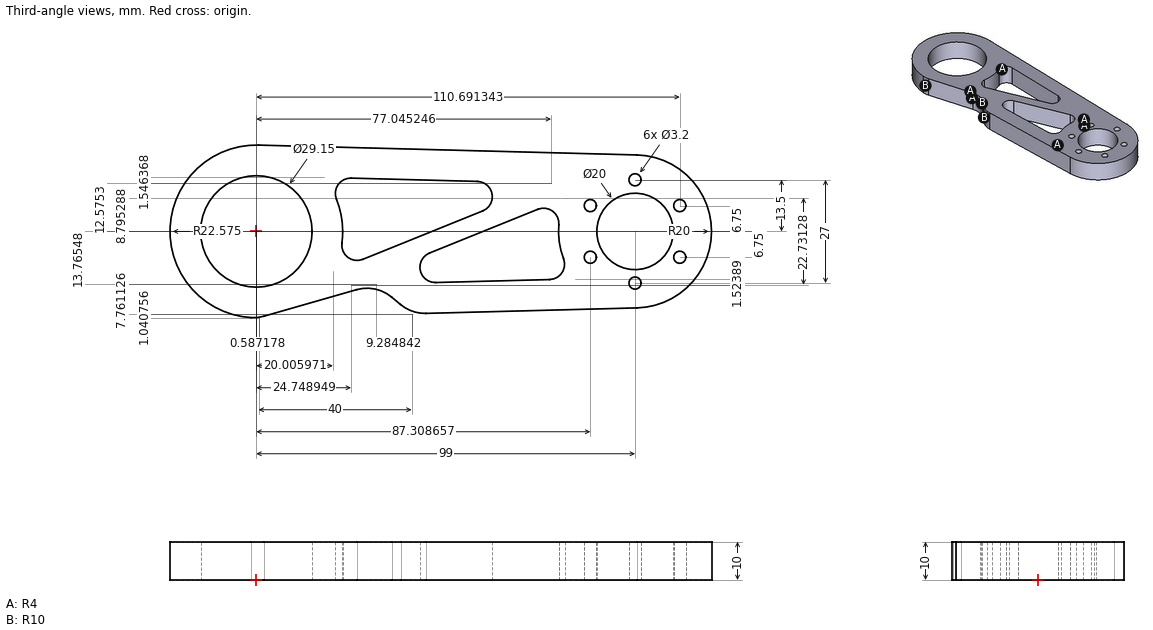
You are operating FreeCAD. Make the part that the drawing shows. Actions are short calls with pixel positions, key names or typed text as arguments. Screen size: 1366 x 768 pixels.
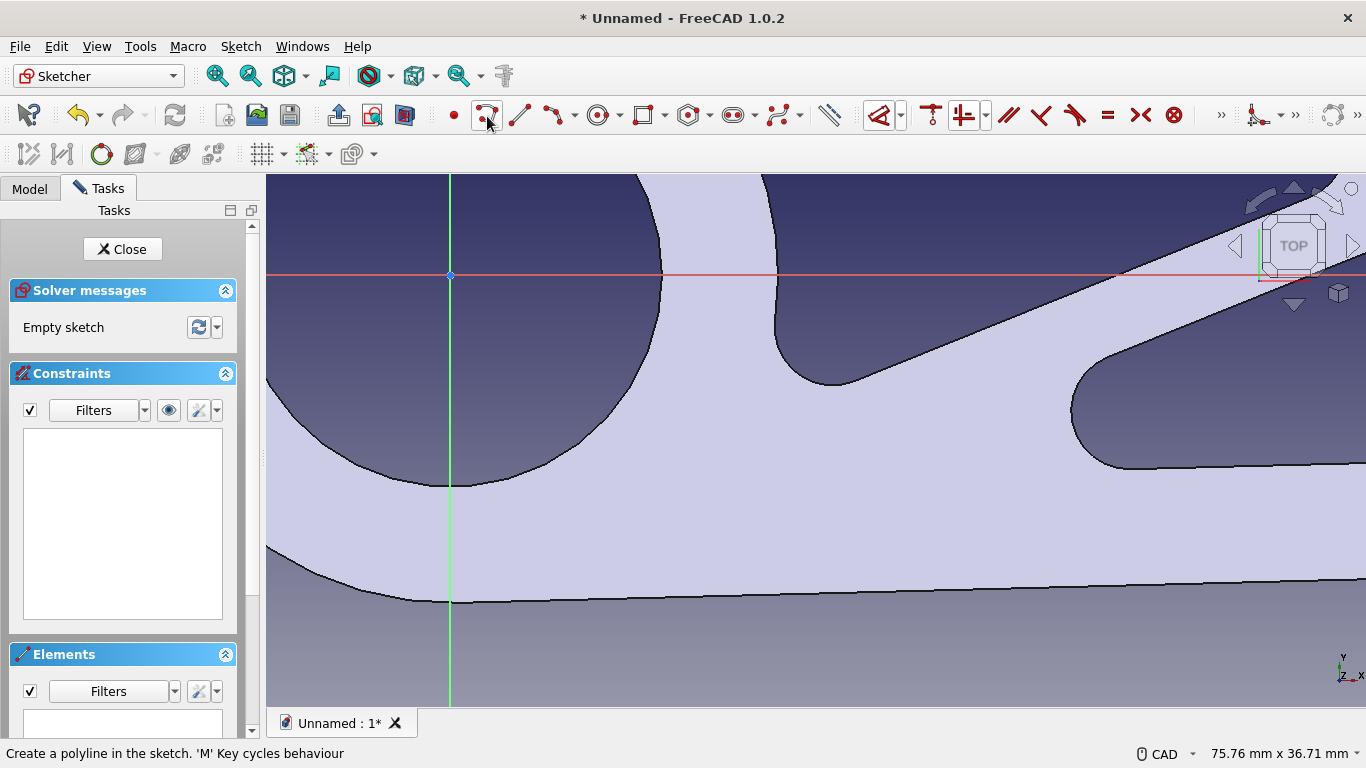
scroll(459, 603, up, 4)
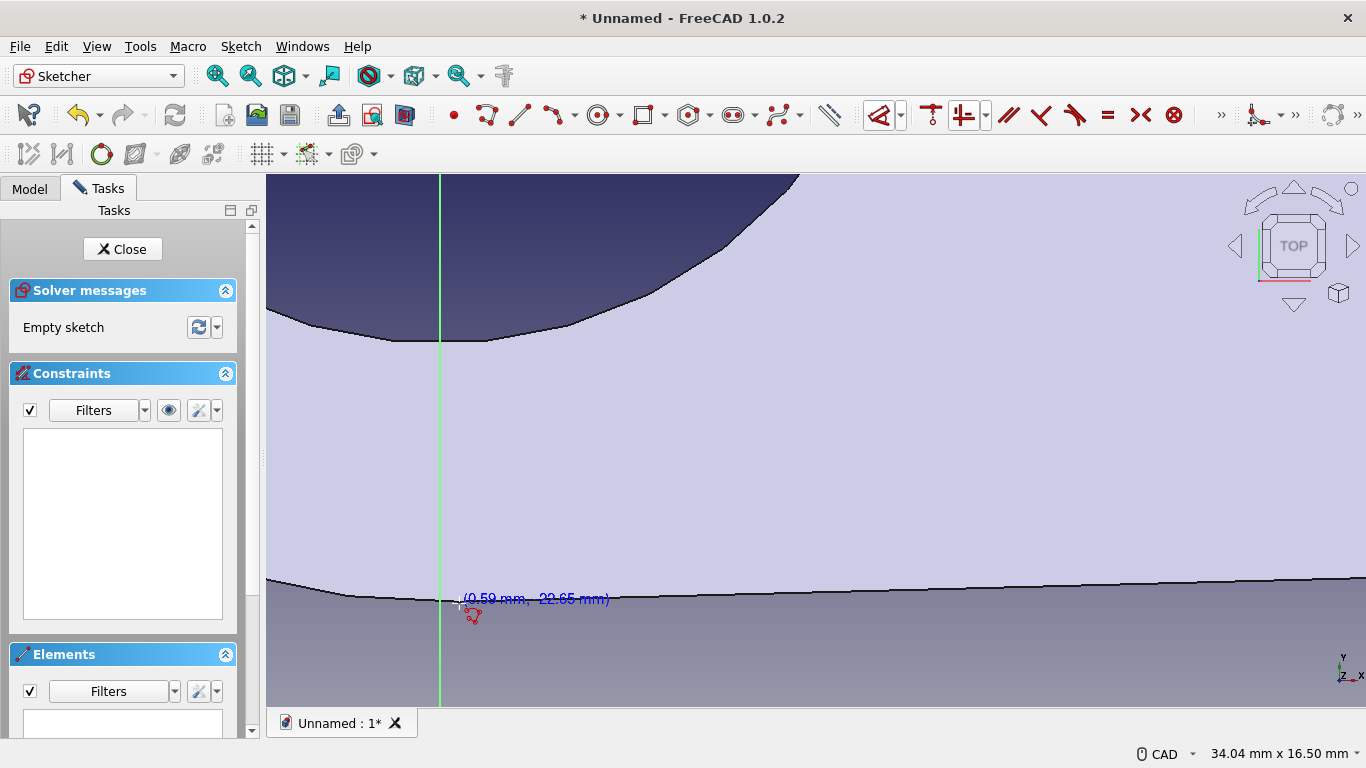
click(459, 602)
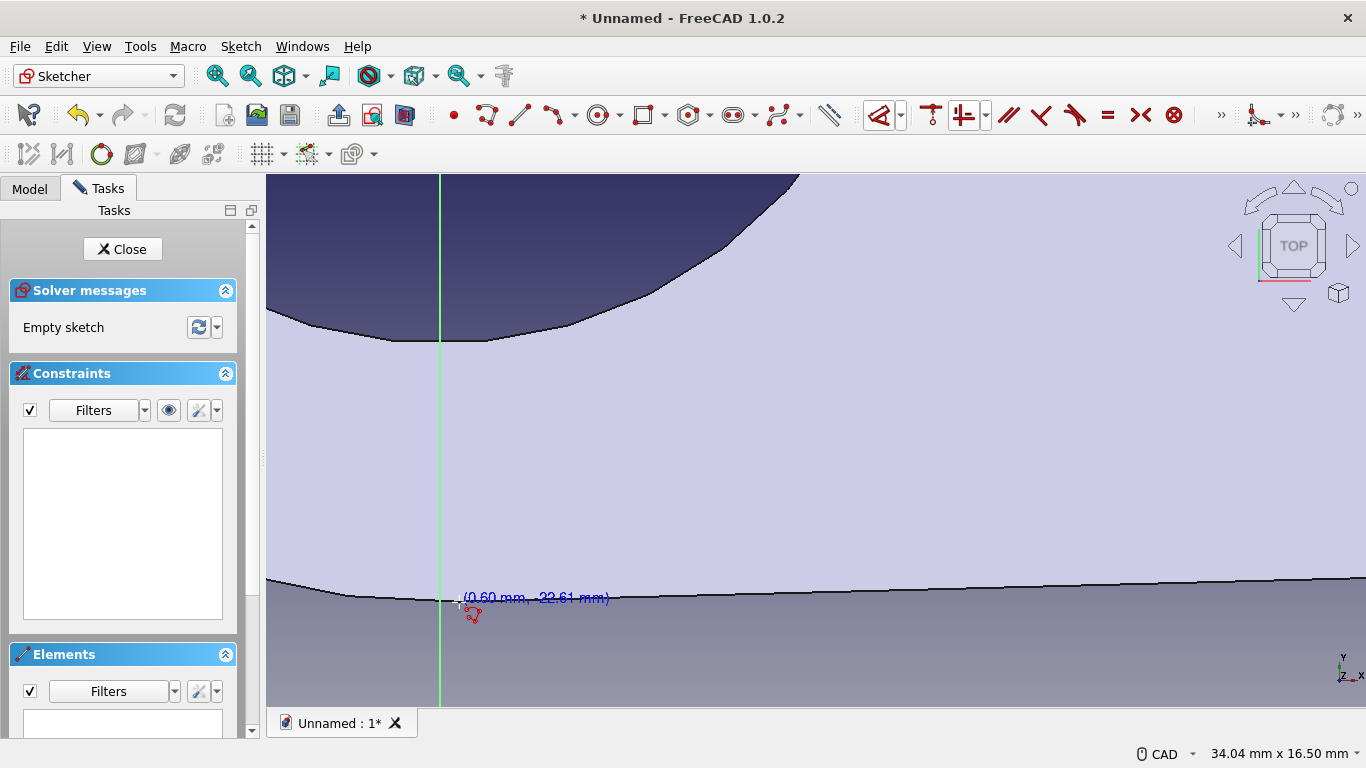
scroll(464, 606, down, 4)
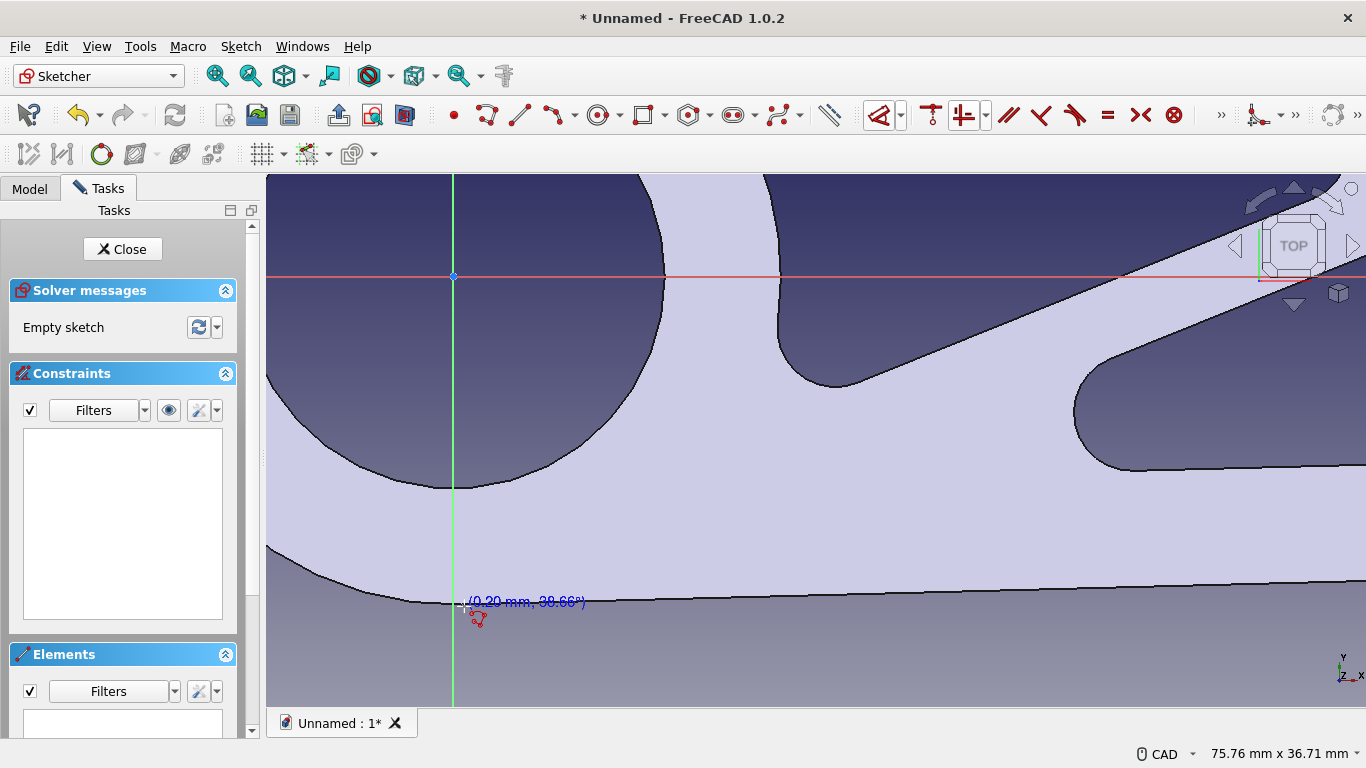
click(1042, 577)
click(908, 477)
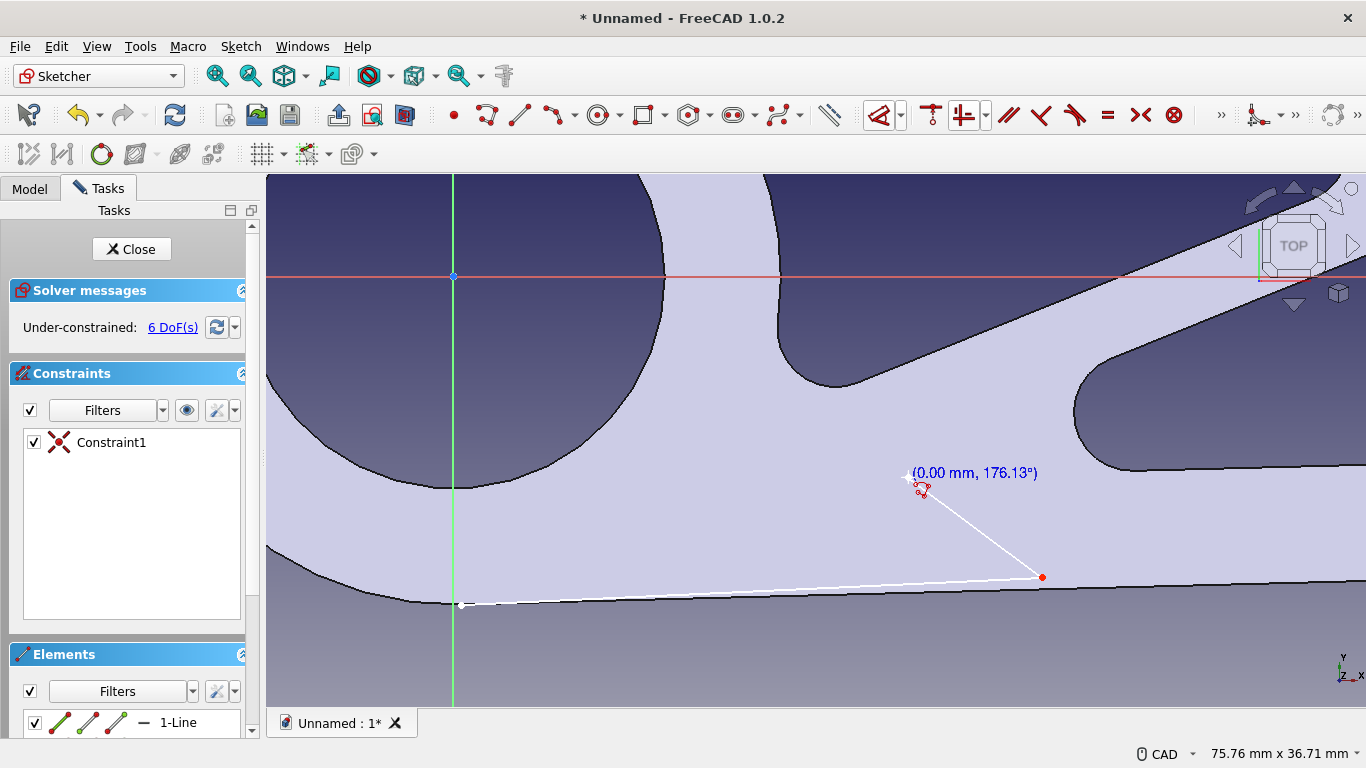
scroll(462, 605, up, 4)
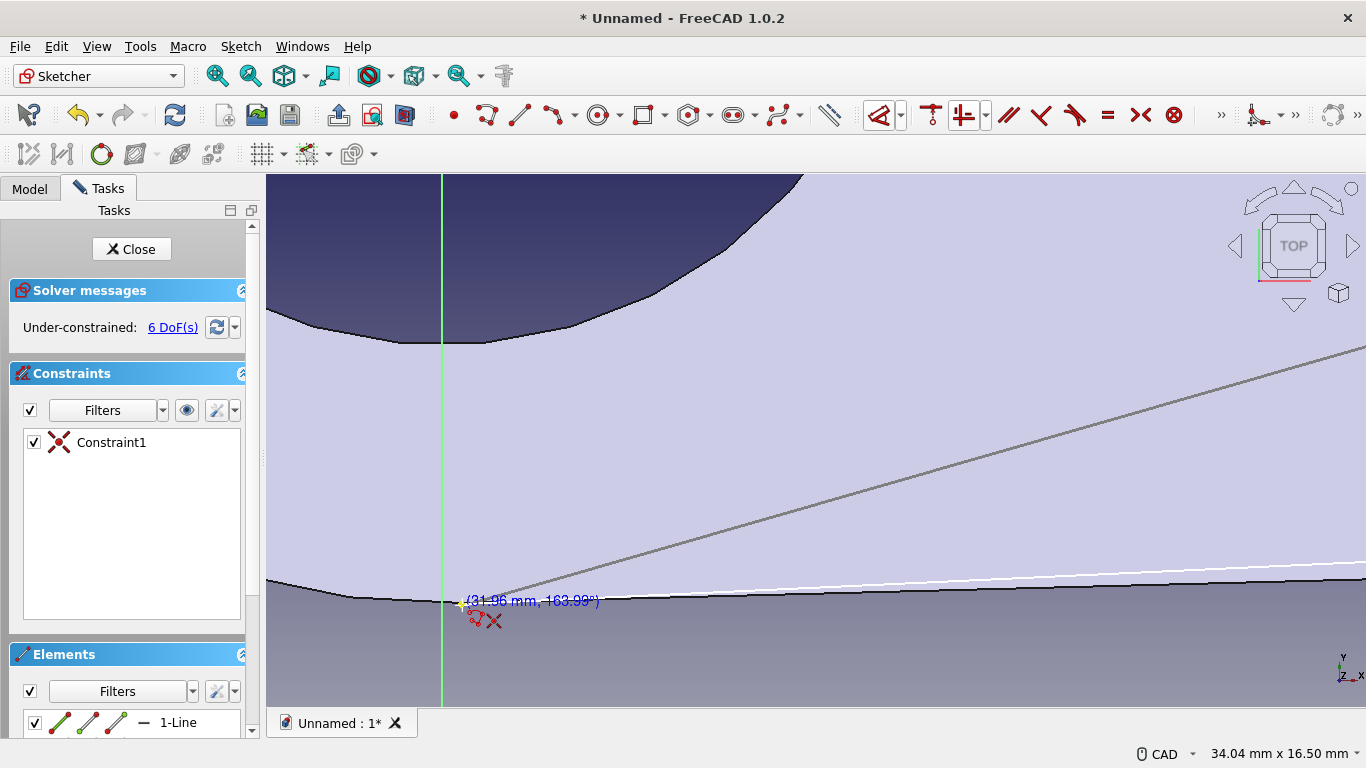
click(461, 604)
key(Escape)
key(Escape)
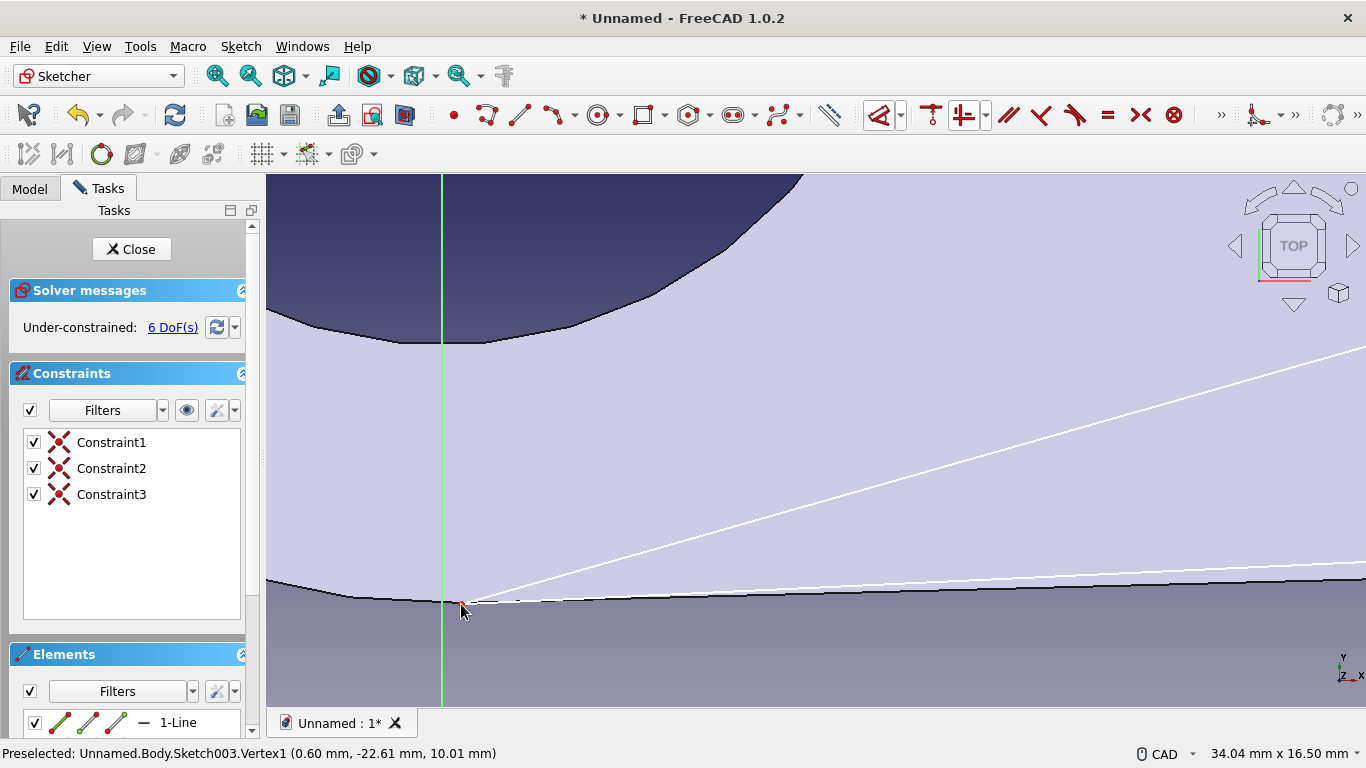
click(849, 586)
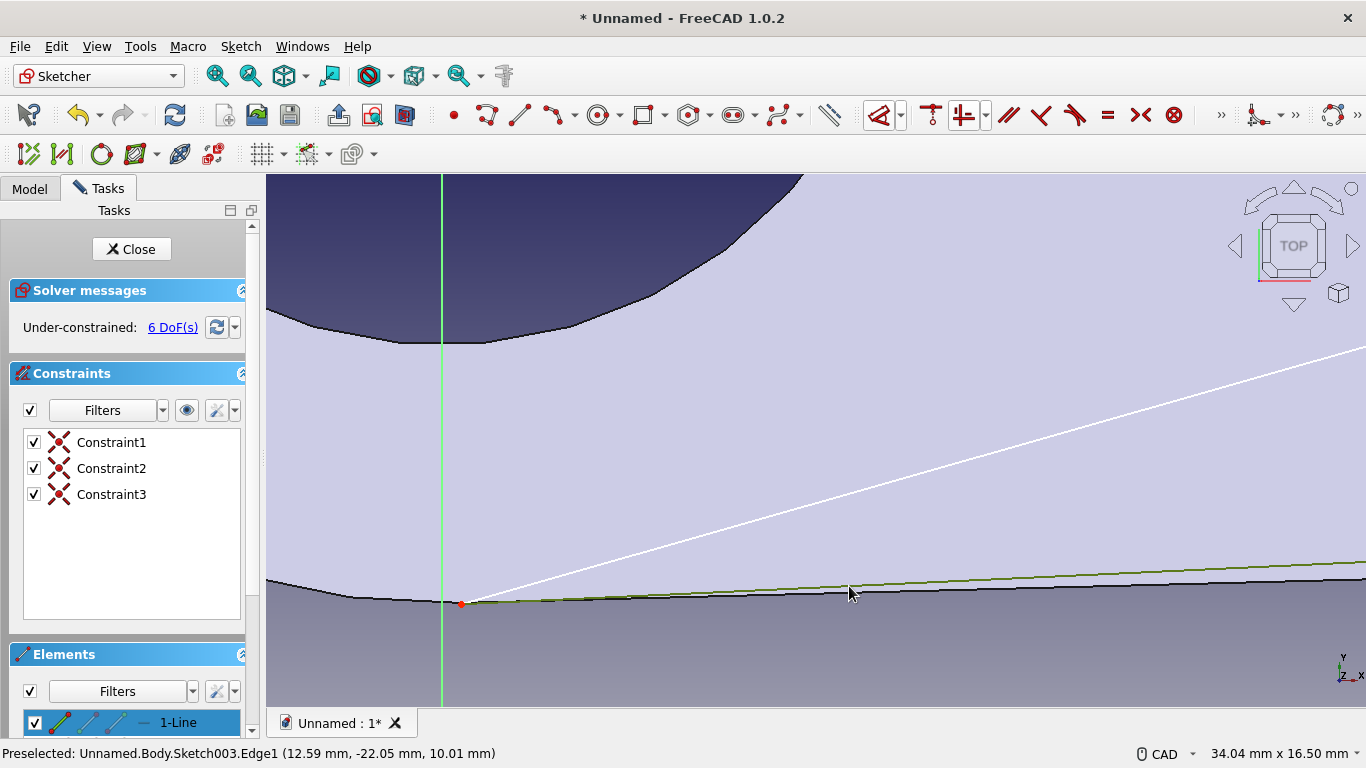
key(l)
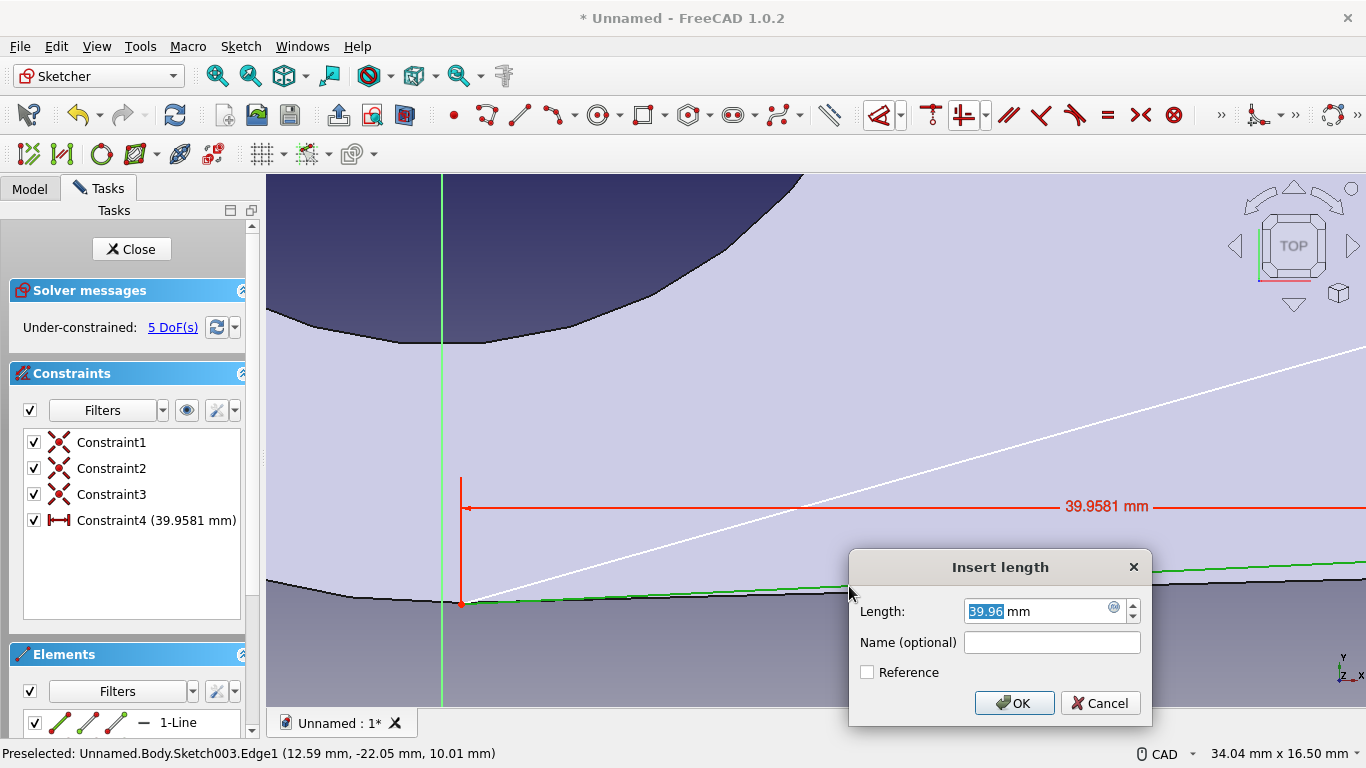
text(40)
key(Return)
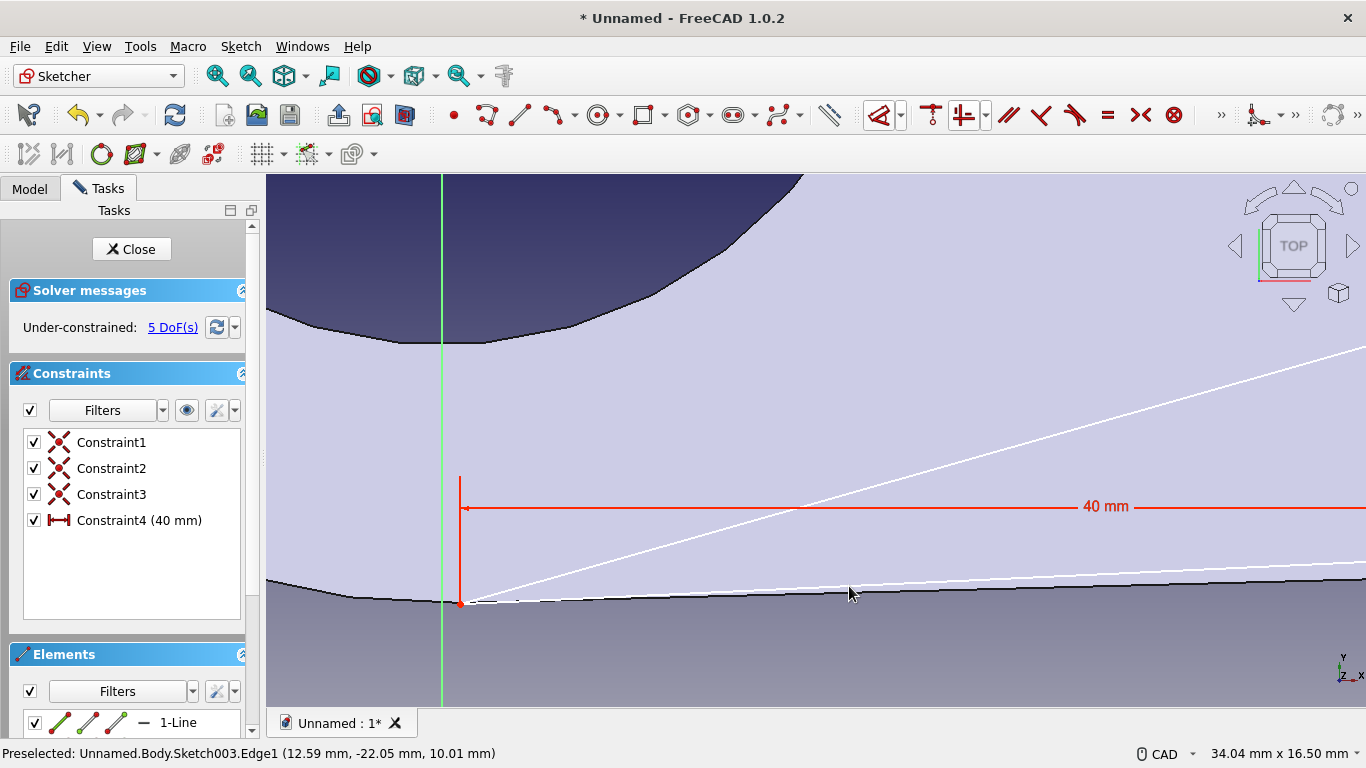
scroll(460, 604, up, 4)